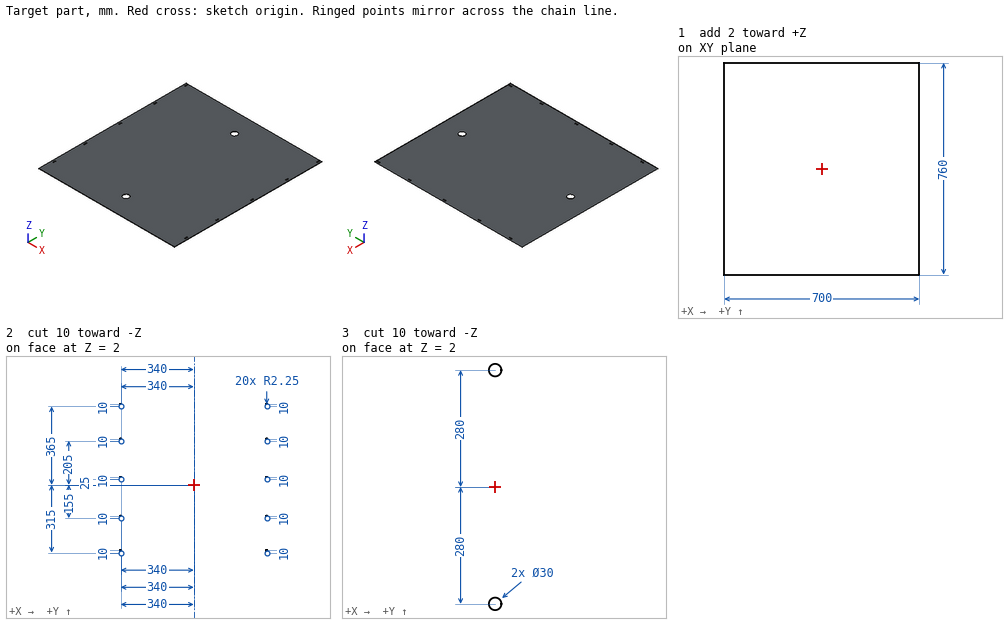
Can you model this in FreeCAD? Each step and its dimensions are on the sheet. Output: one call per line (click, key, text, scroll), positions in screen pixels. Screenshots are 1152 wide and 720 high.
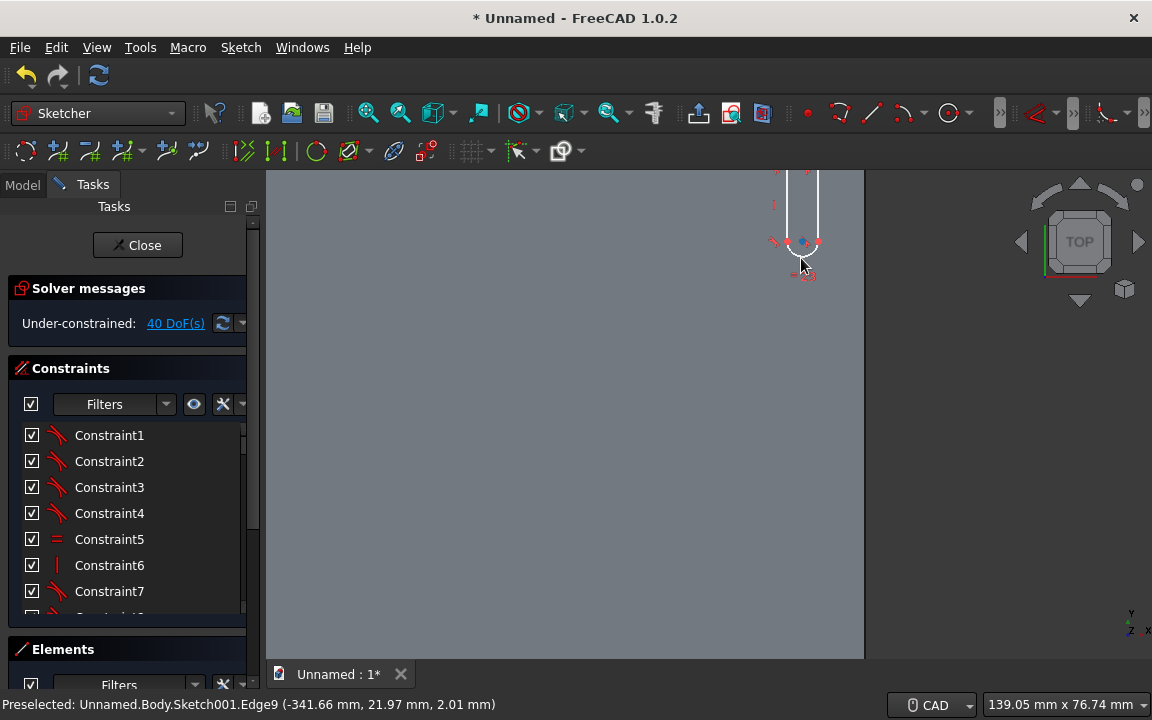
click(793, 254)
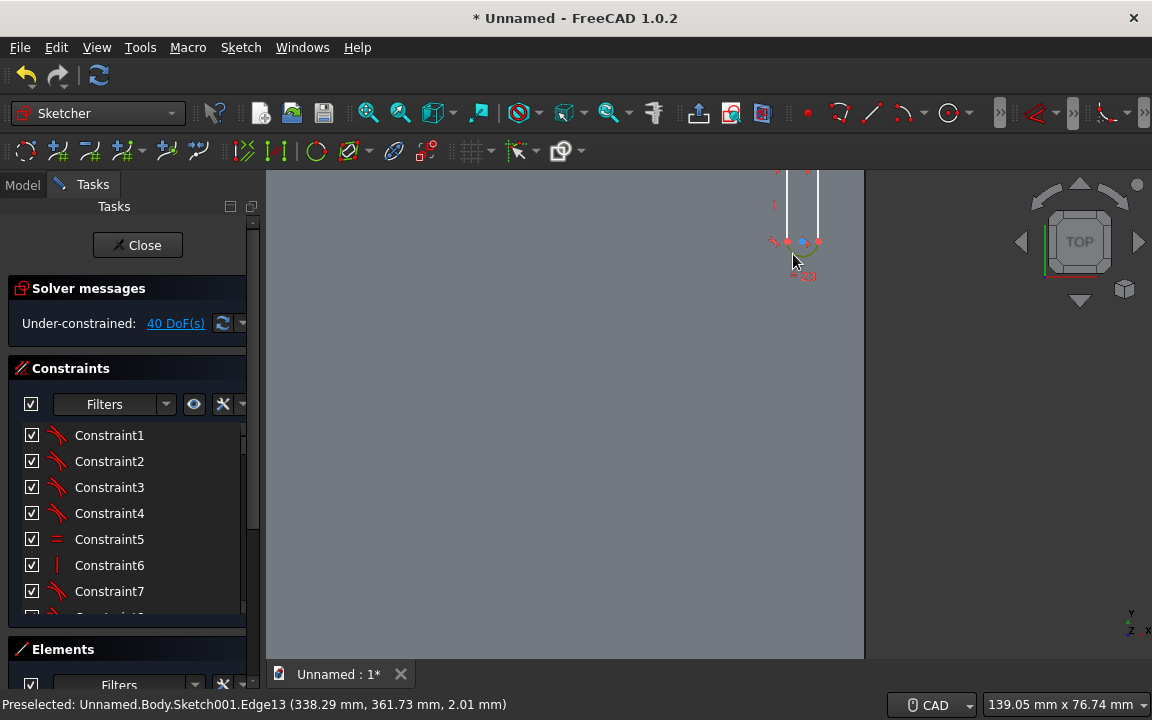
scroll(801, 258, down, 13)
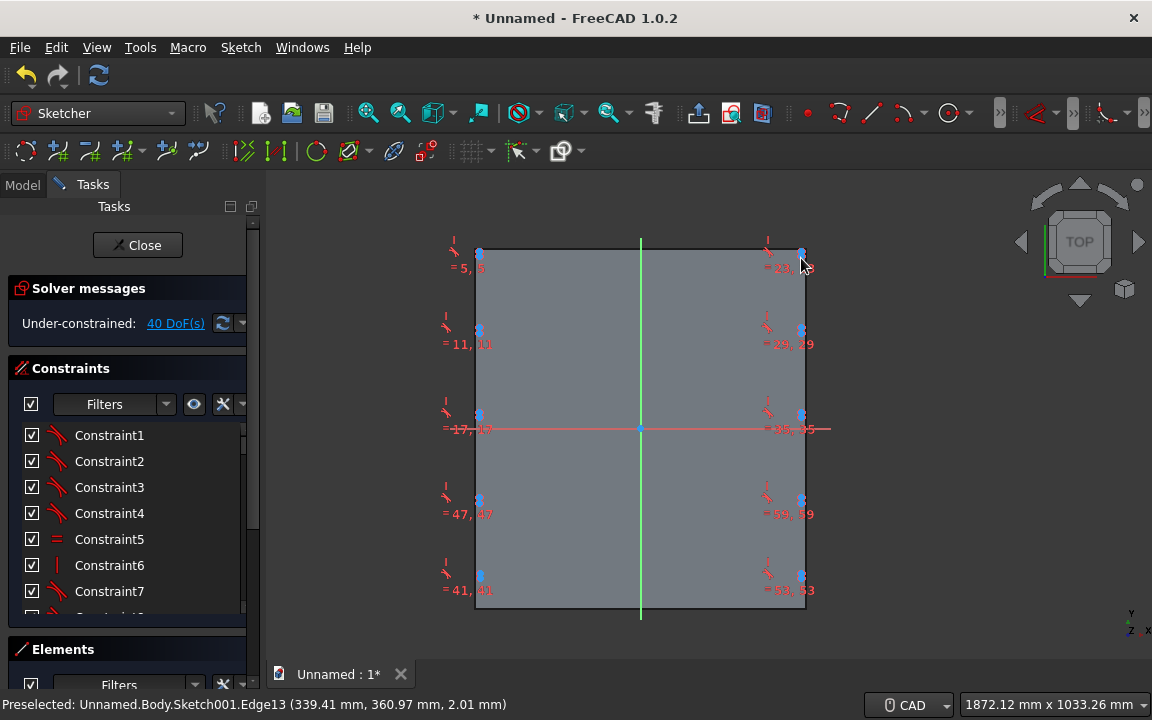
scroll(801, 334, up, 13)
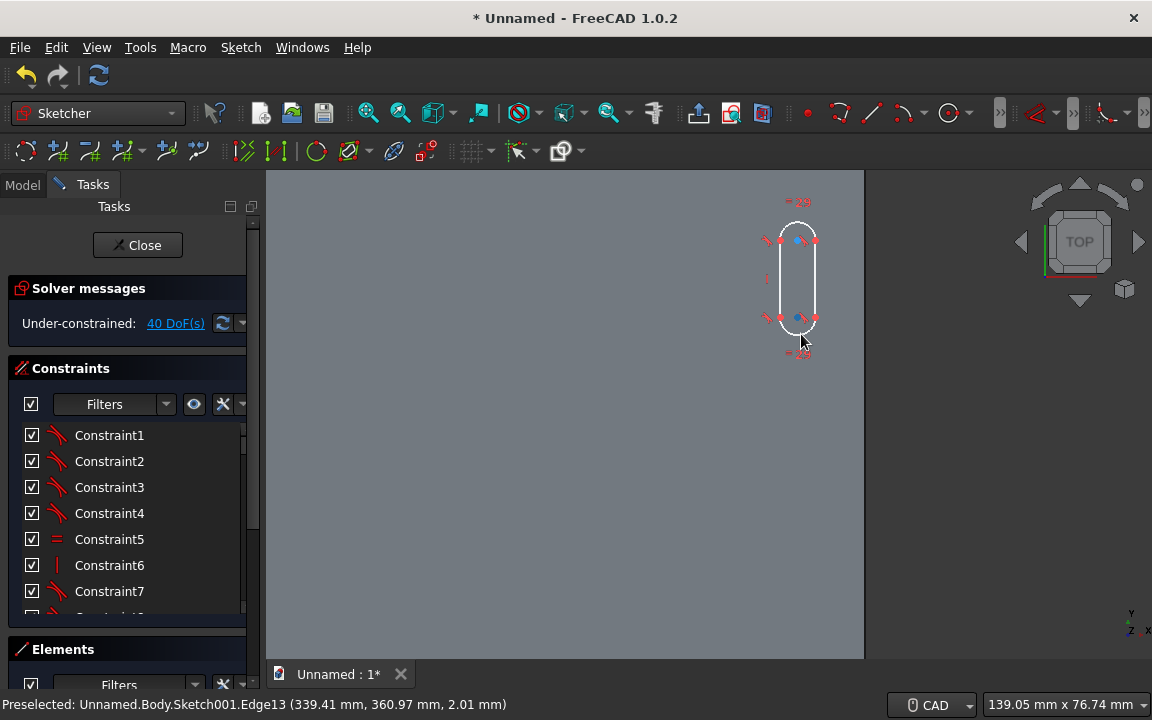
click(787, 332)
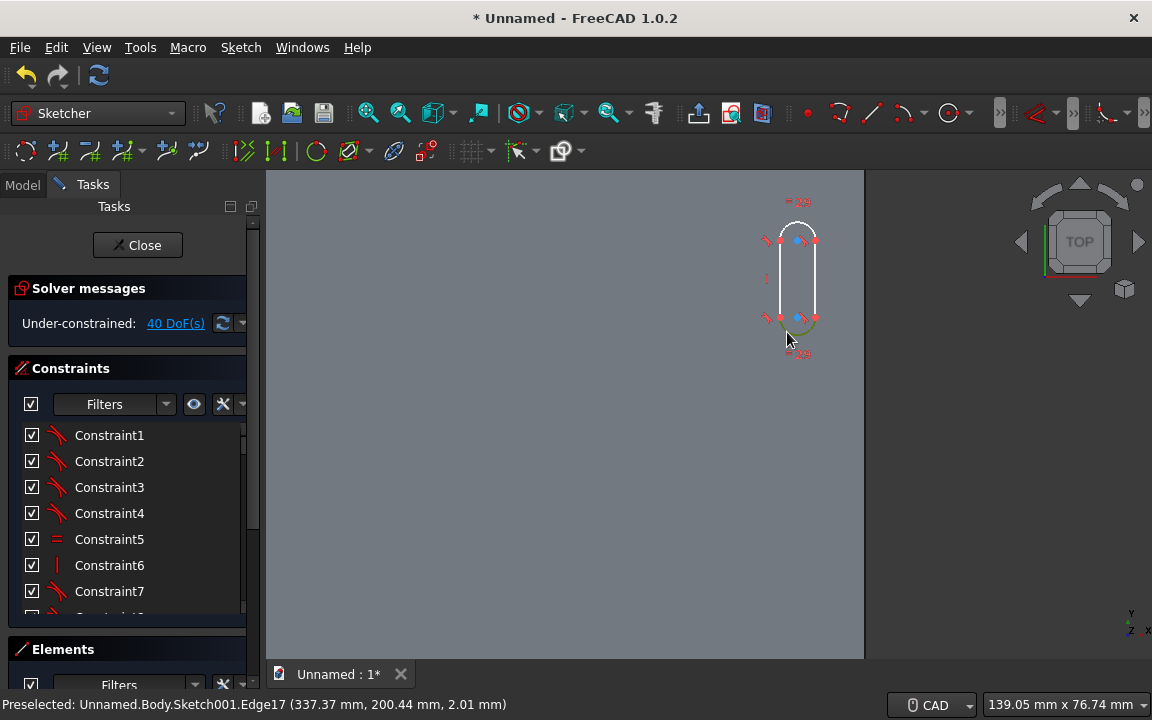
scroll(801, 334, down, 13)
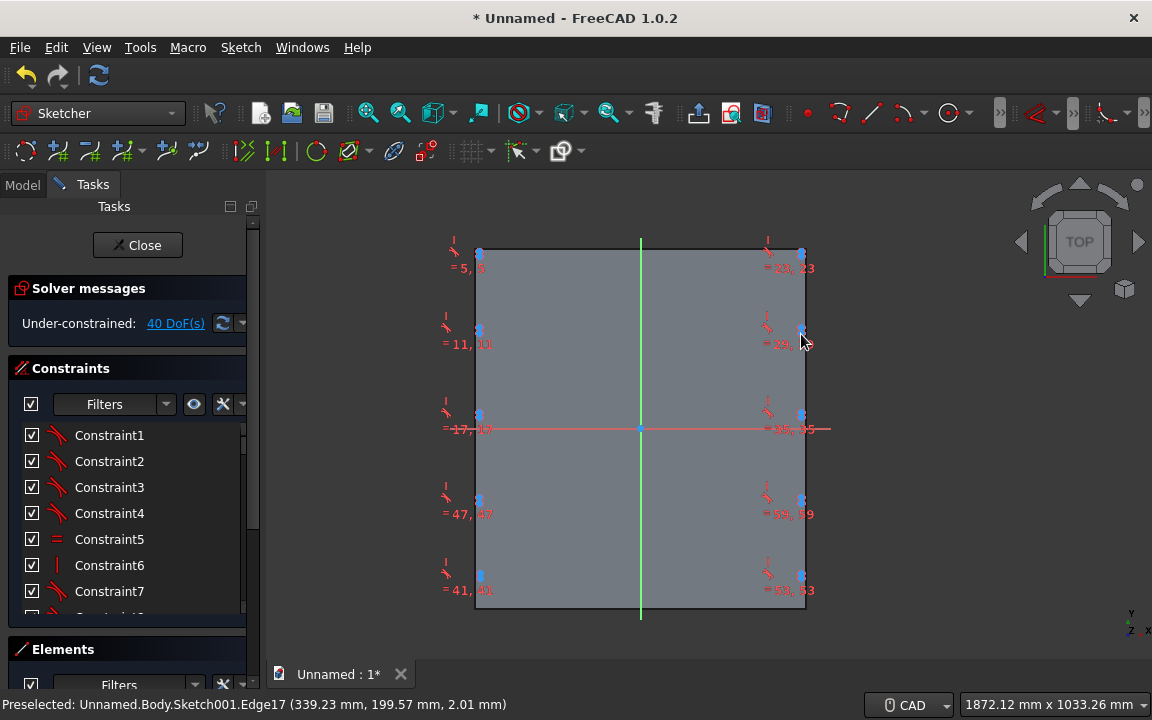
scroll(801, 419, up, 14)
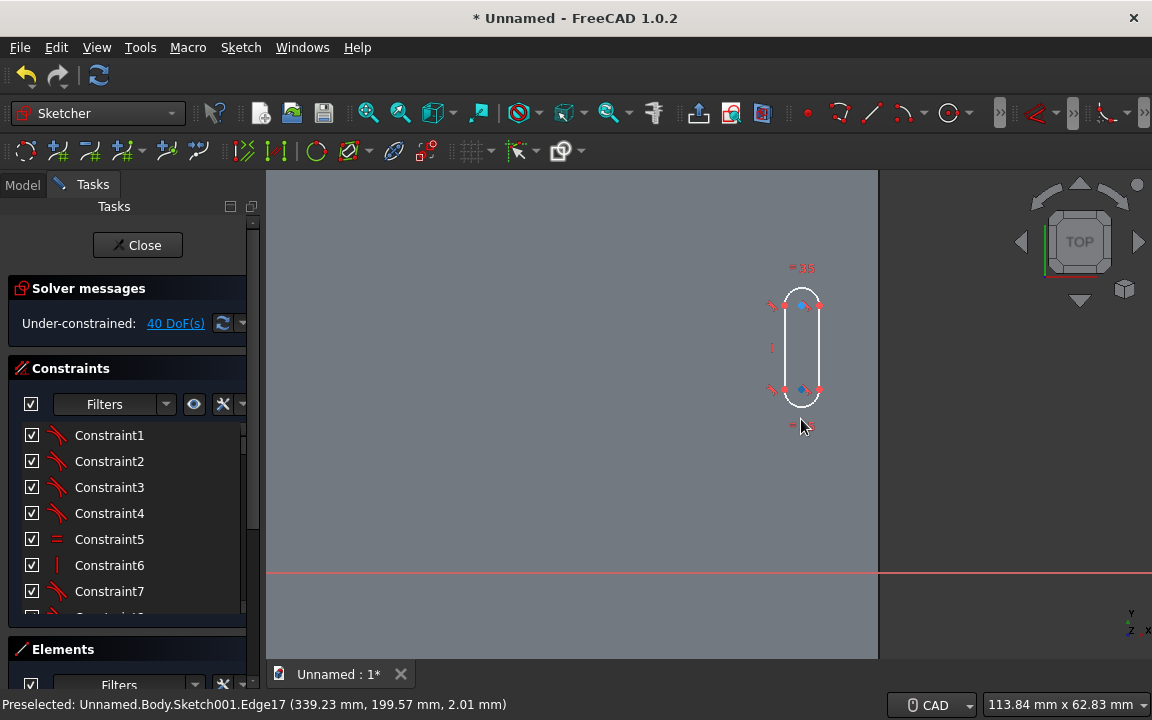
click(792, 404)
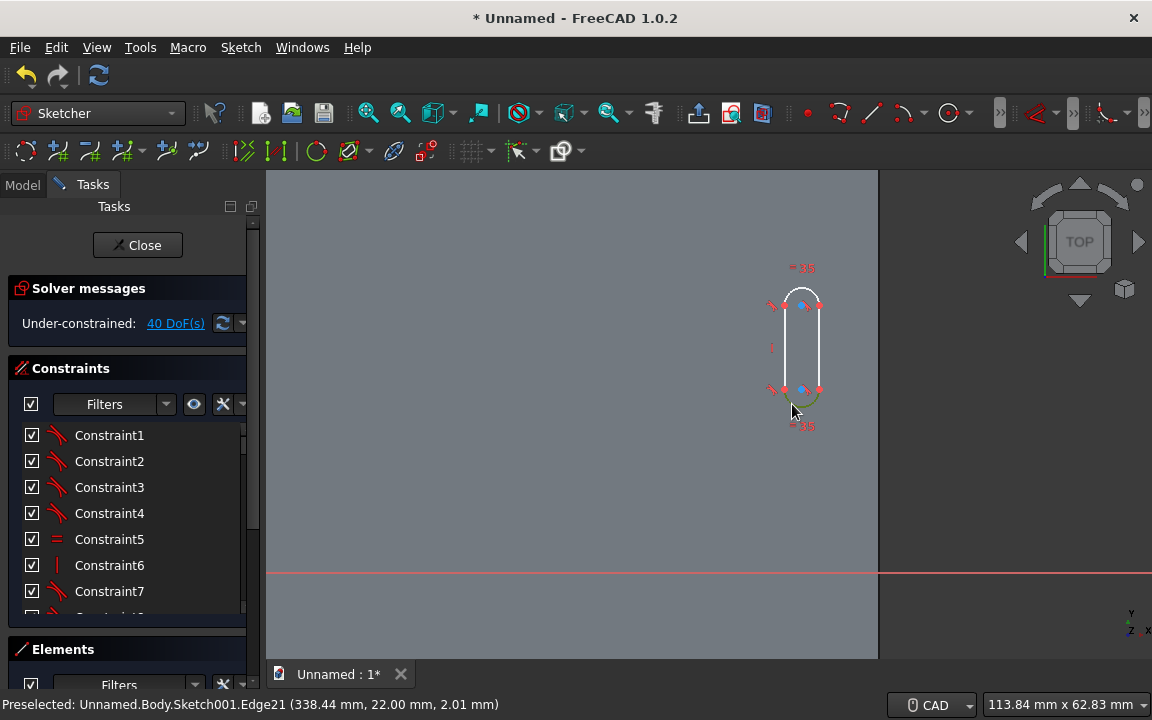
scroll(801, 419, down, 14)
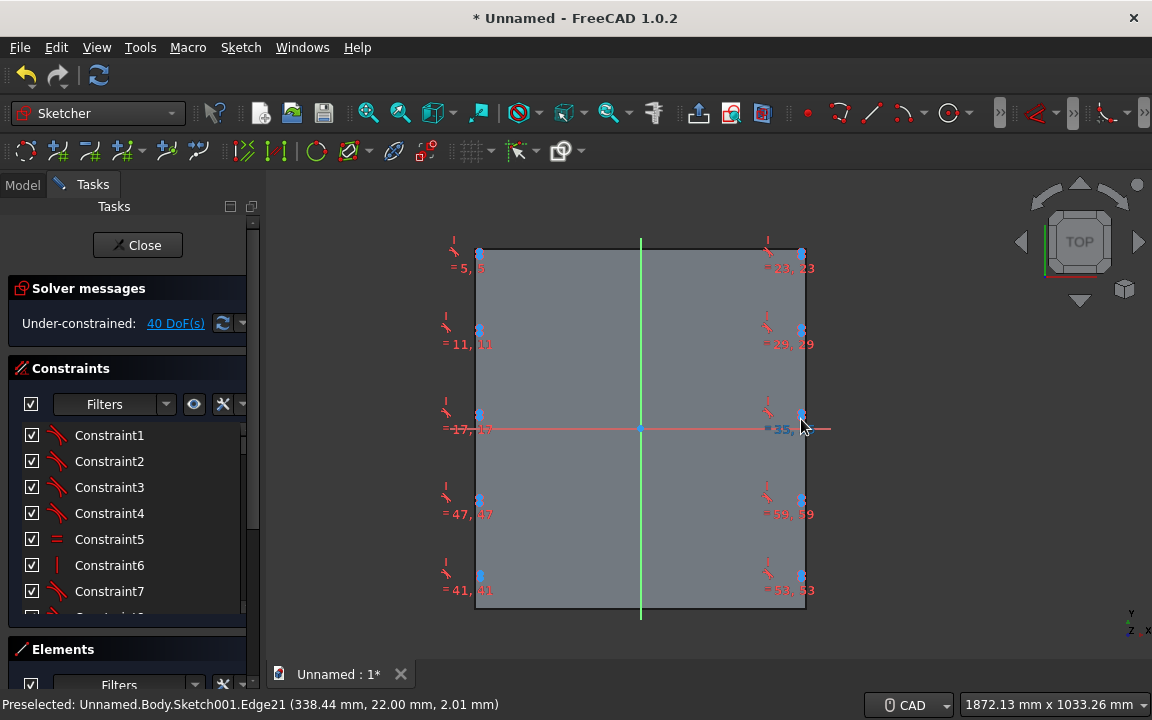
scroll(479, 580, up, 14)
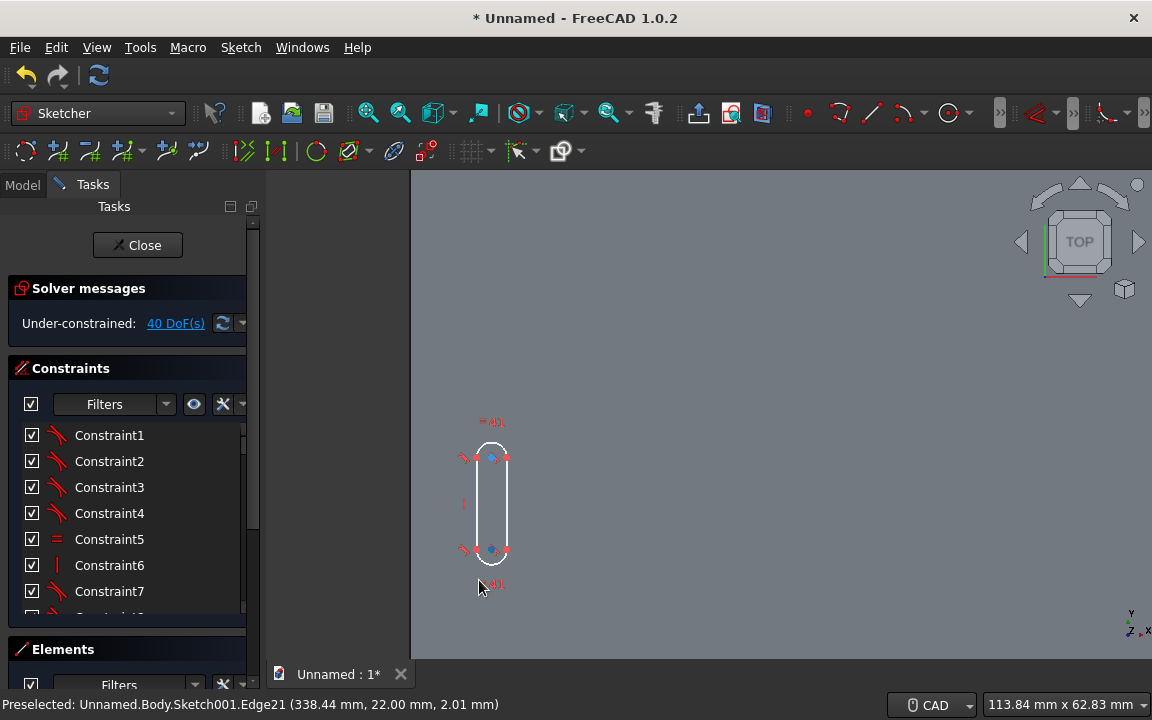
click(483, 562)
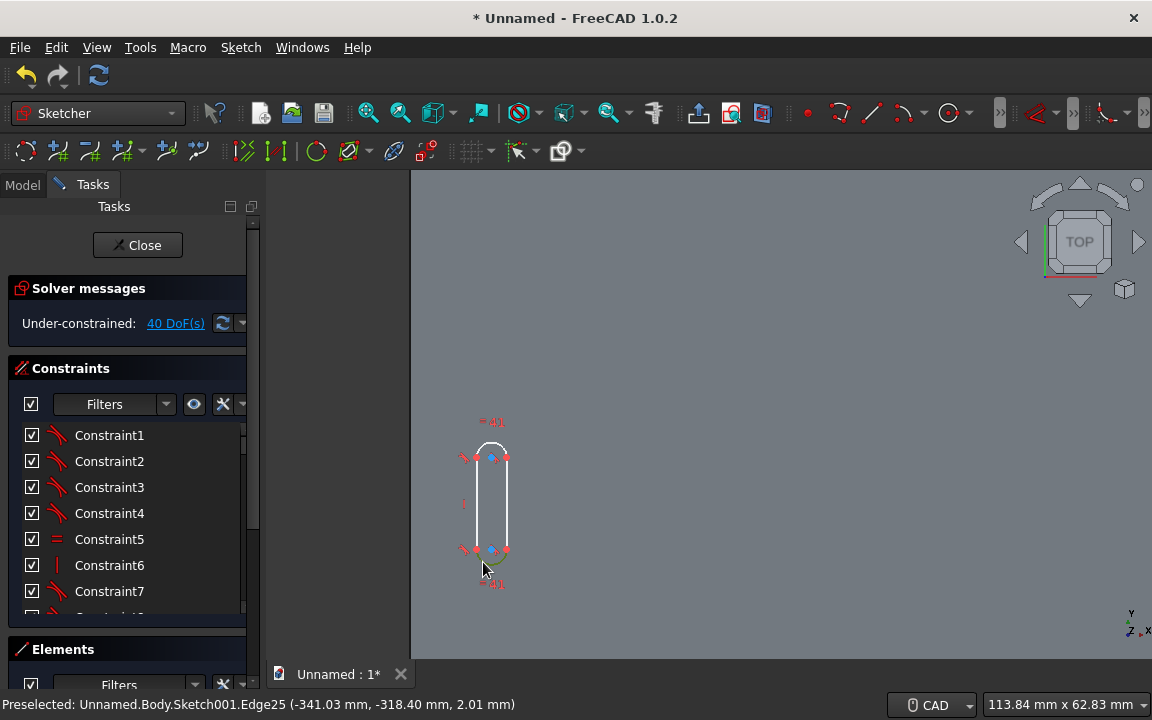
scroll(479, 581, down, 14)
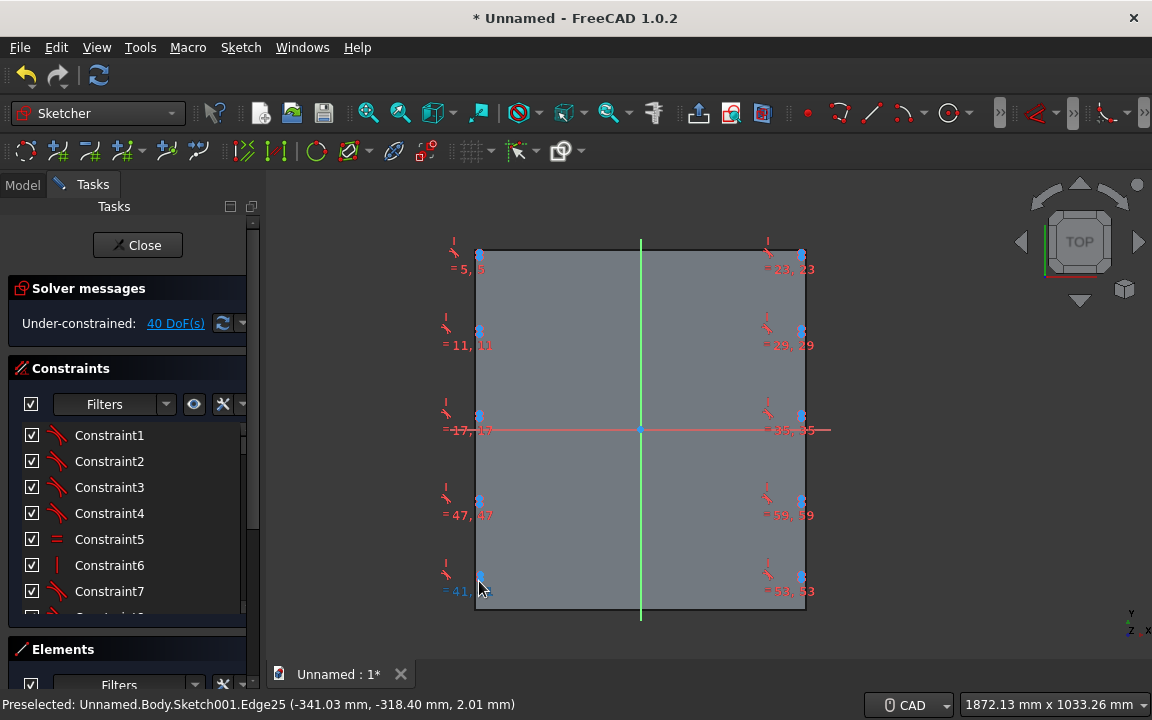
scroll(479, 505, up, 13)